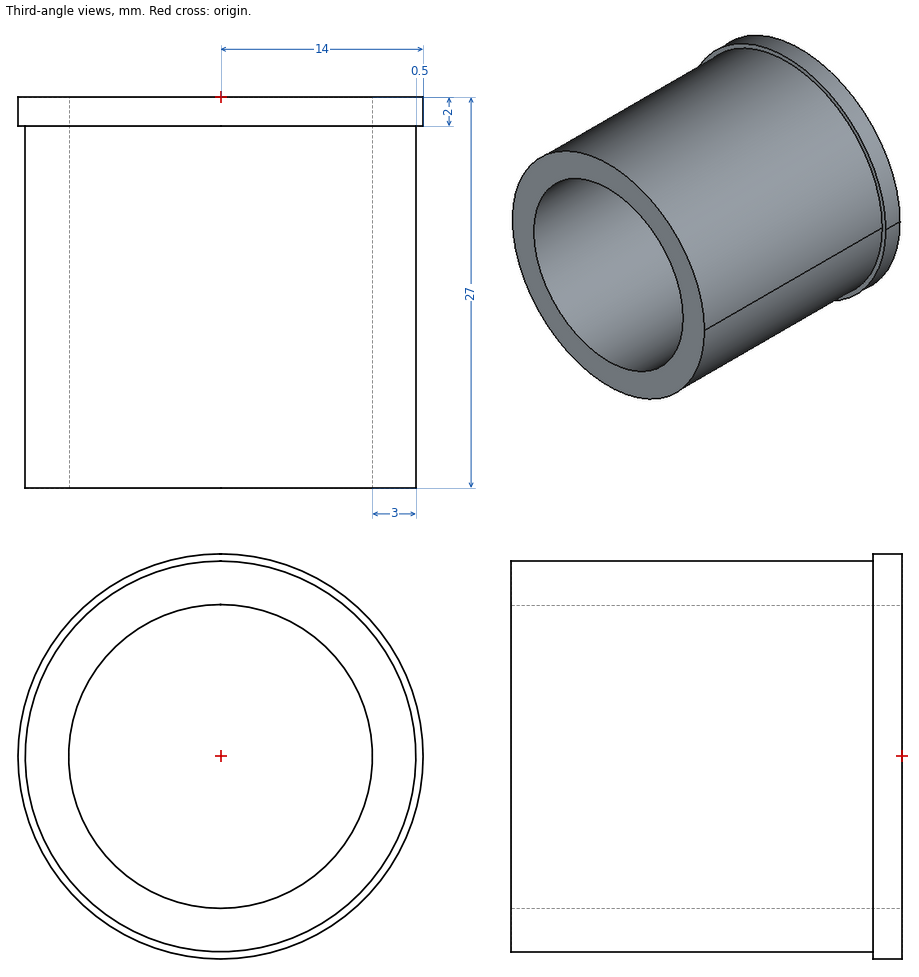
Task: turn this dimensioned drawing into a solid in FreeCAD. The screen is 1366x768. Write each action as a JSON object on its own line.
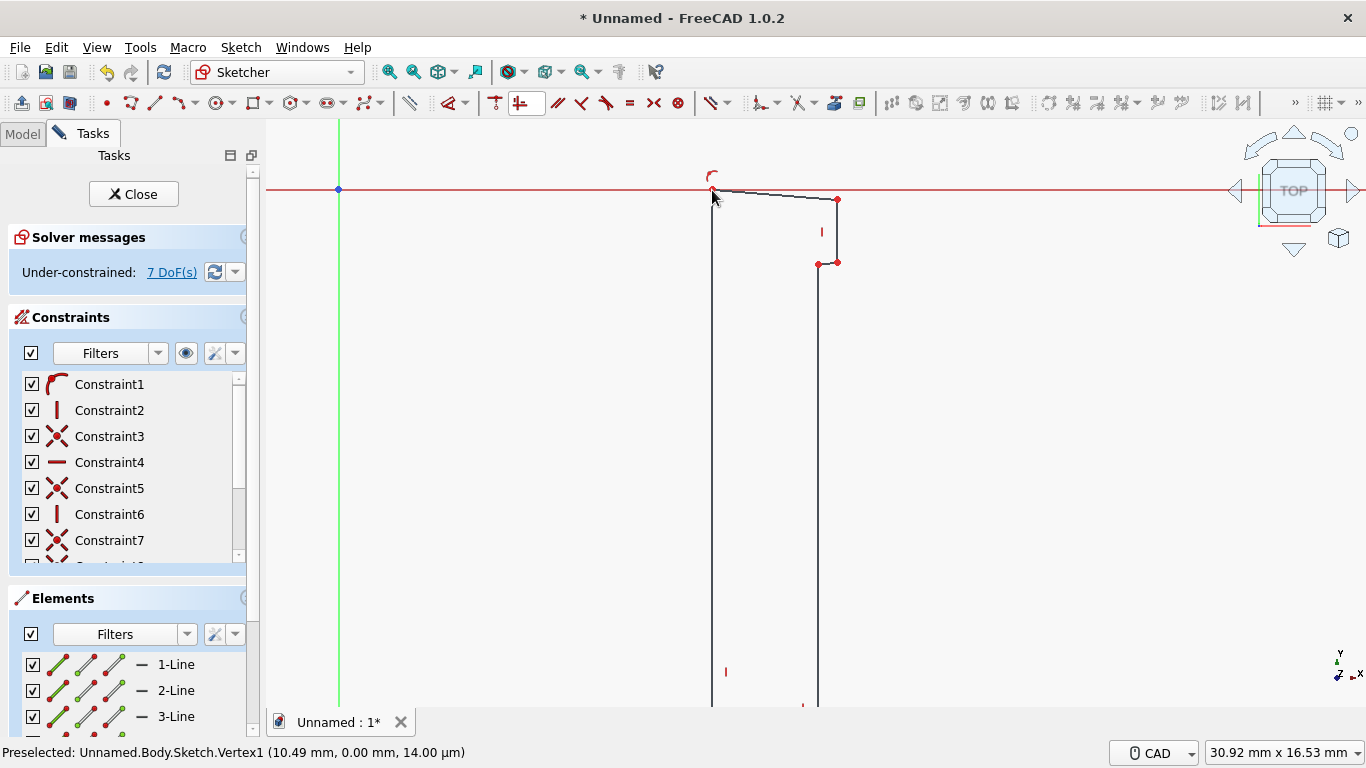
{"action": "scroll", "coordinate": [828, 264], "scroll_direction": "up", "scroll_amount": 2}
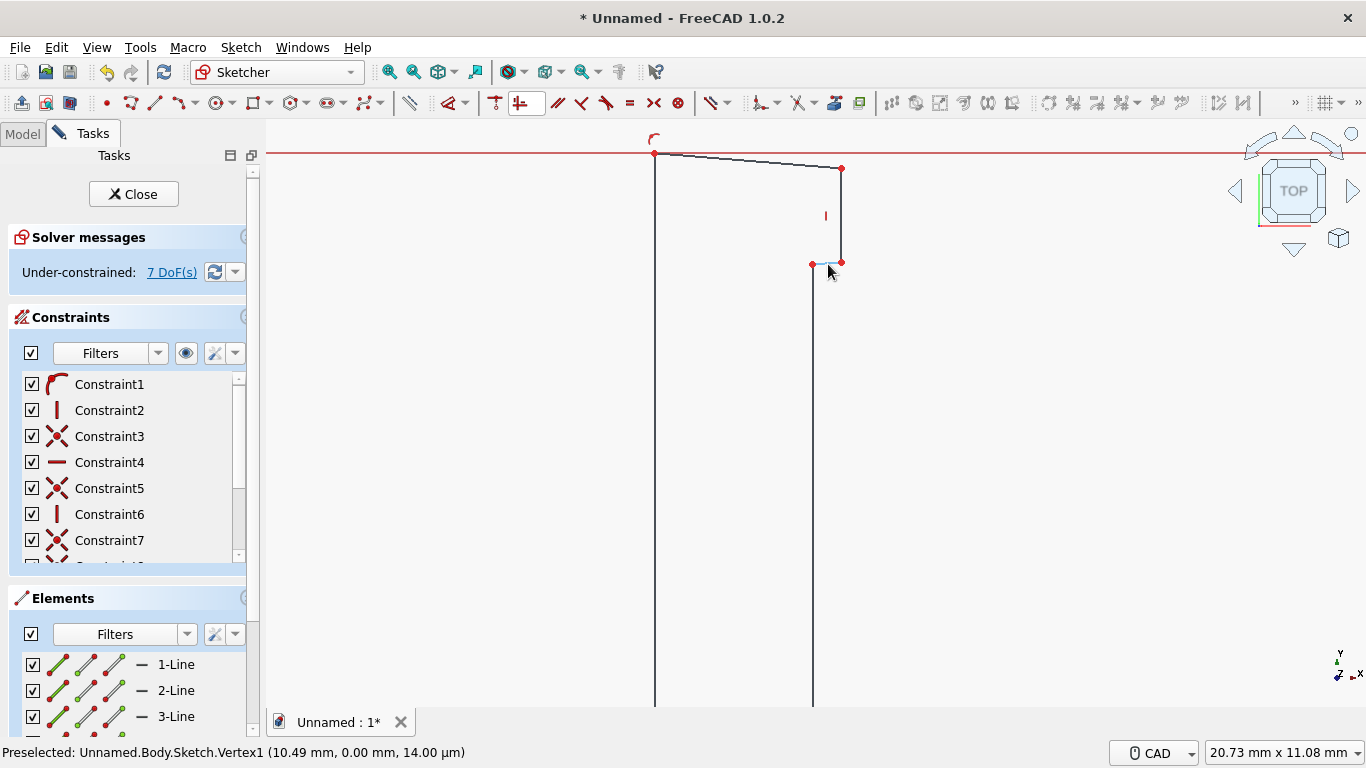
{"action": "left_click", "coordinate": [827, 263]}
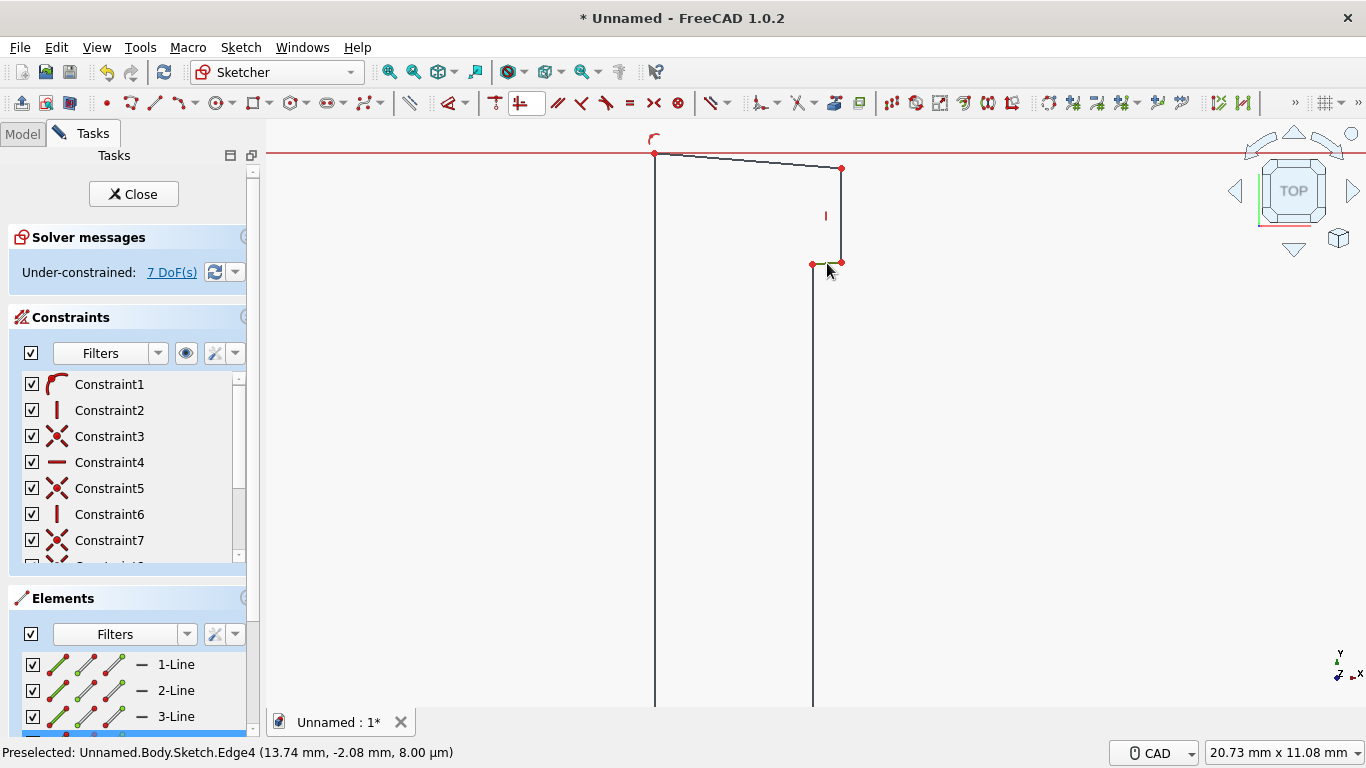
{"action": "key", "text": "h"}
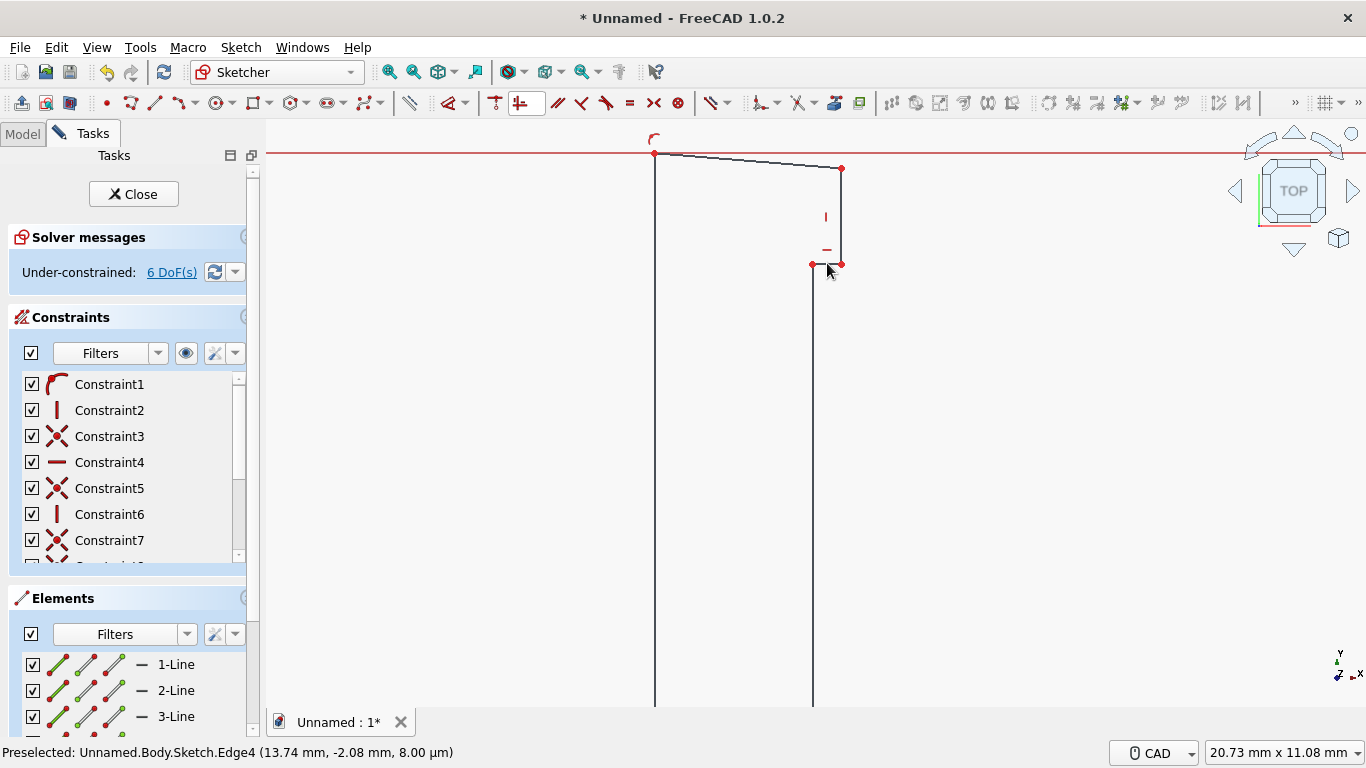
{"action": "scroll", "coordinate": [785, 164], "scroll_direction": "up", "scroll_amount": 2}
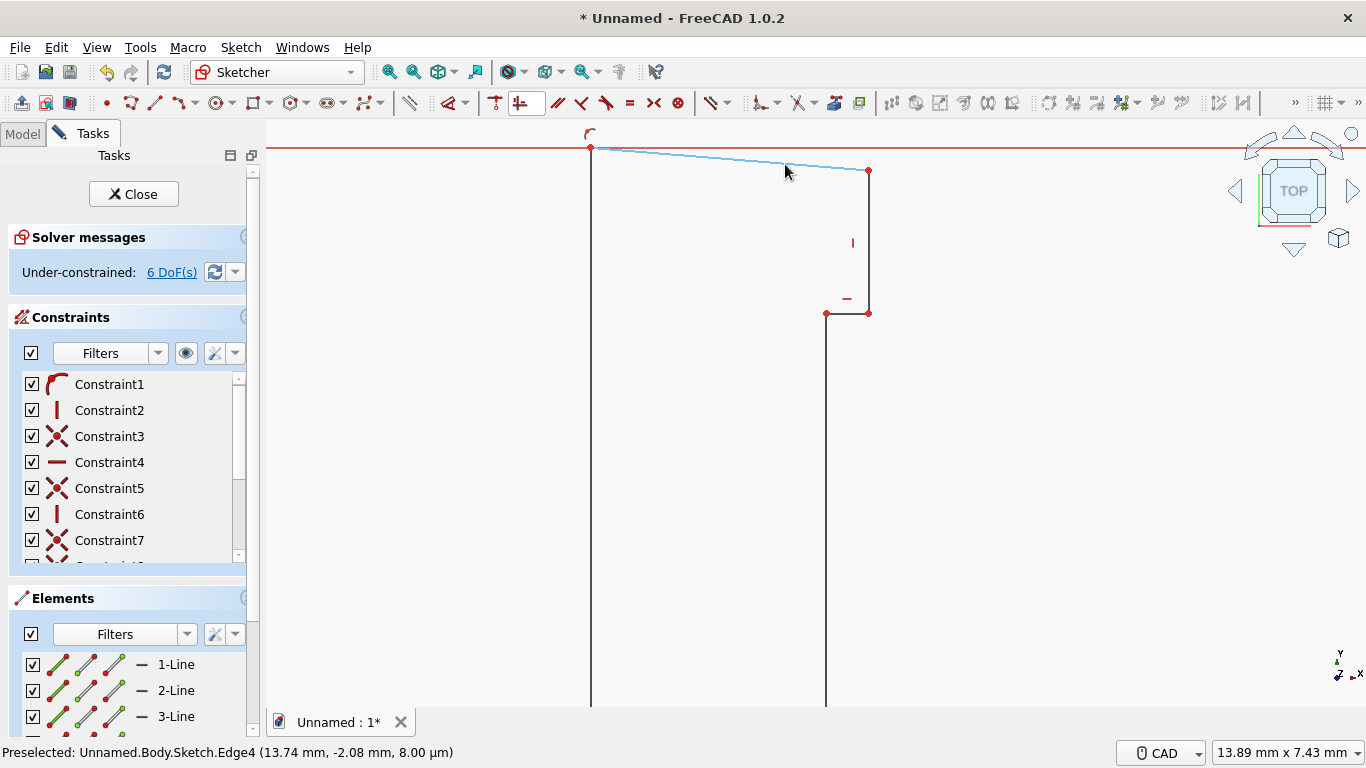
{"action": "left_click", "coordinate": [785, 164]}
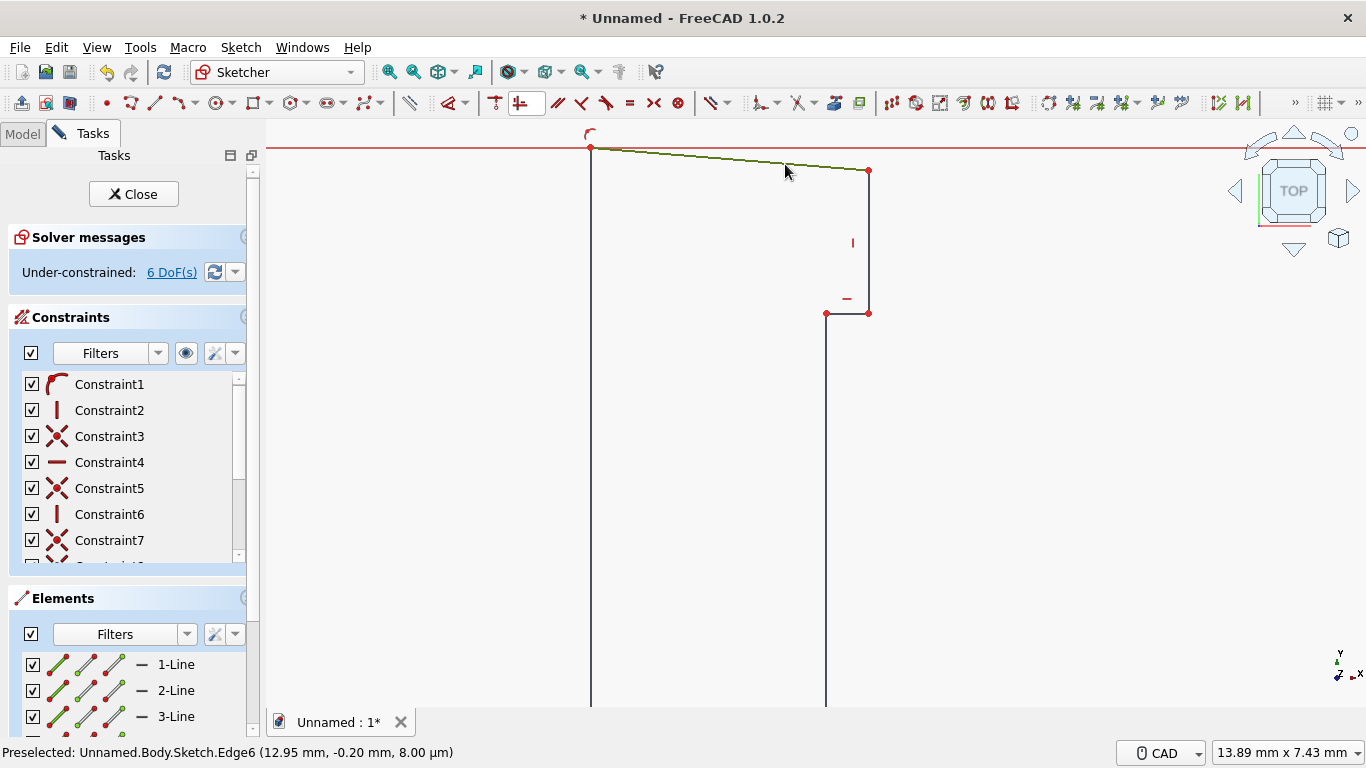
{"action": "key", "text": "h"}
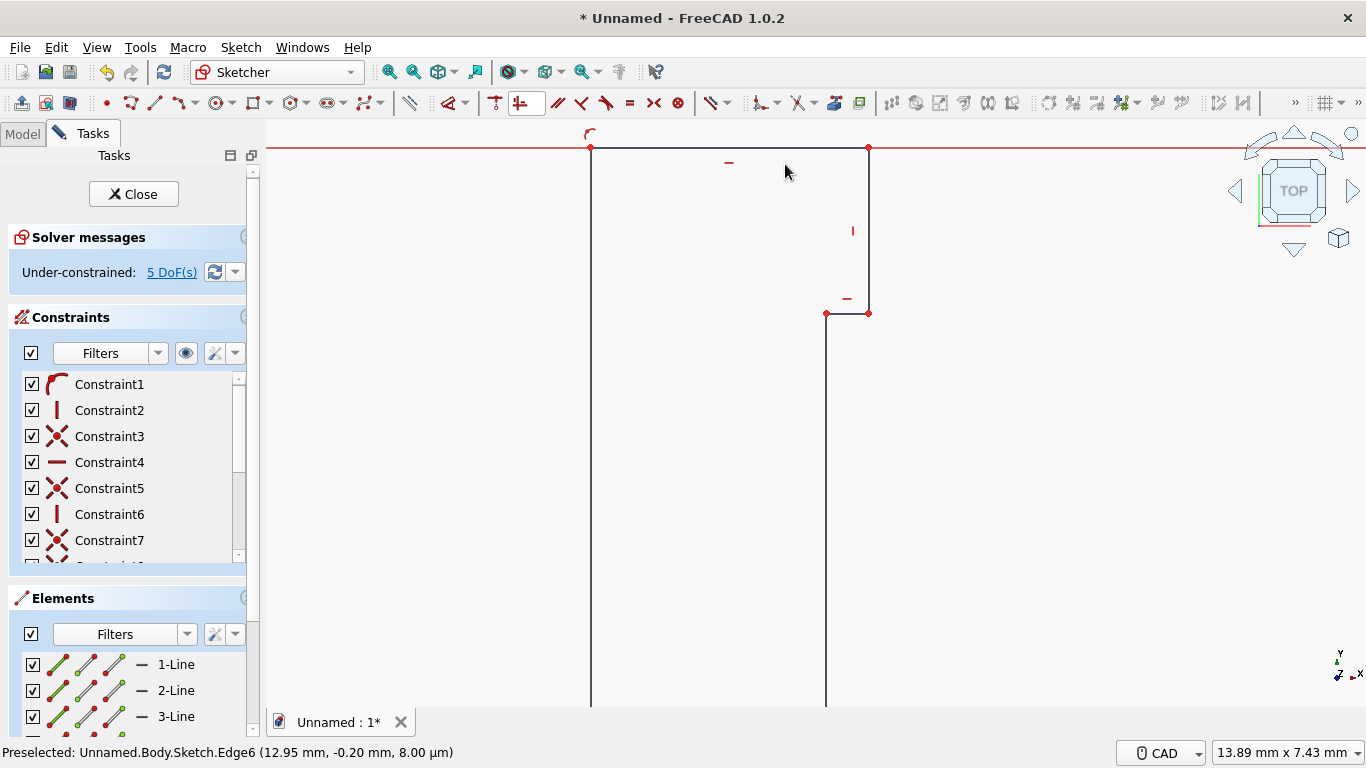
{"action": "scroll", "coordinate": [833, 254], "scroll_direction": "down", "scroll_amount": 9}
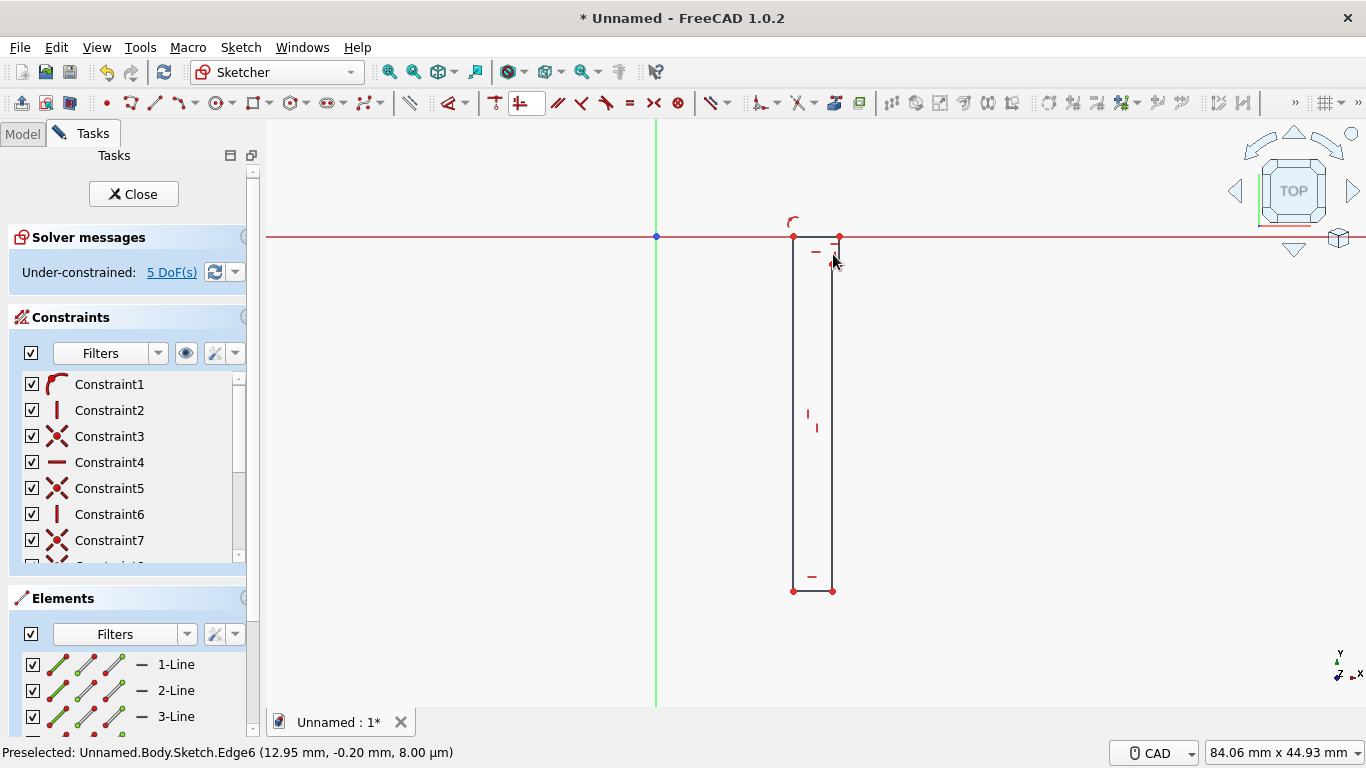
{"action": "left_click", "coordinate": [805, 591]}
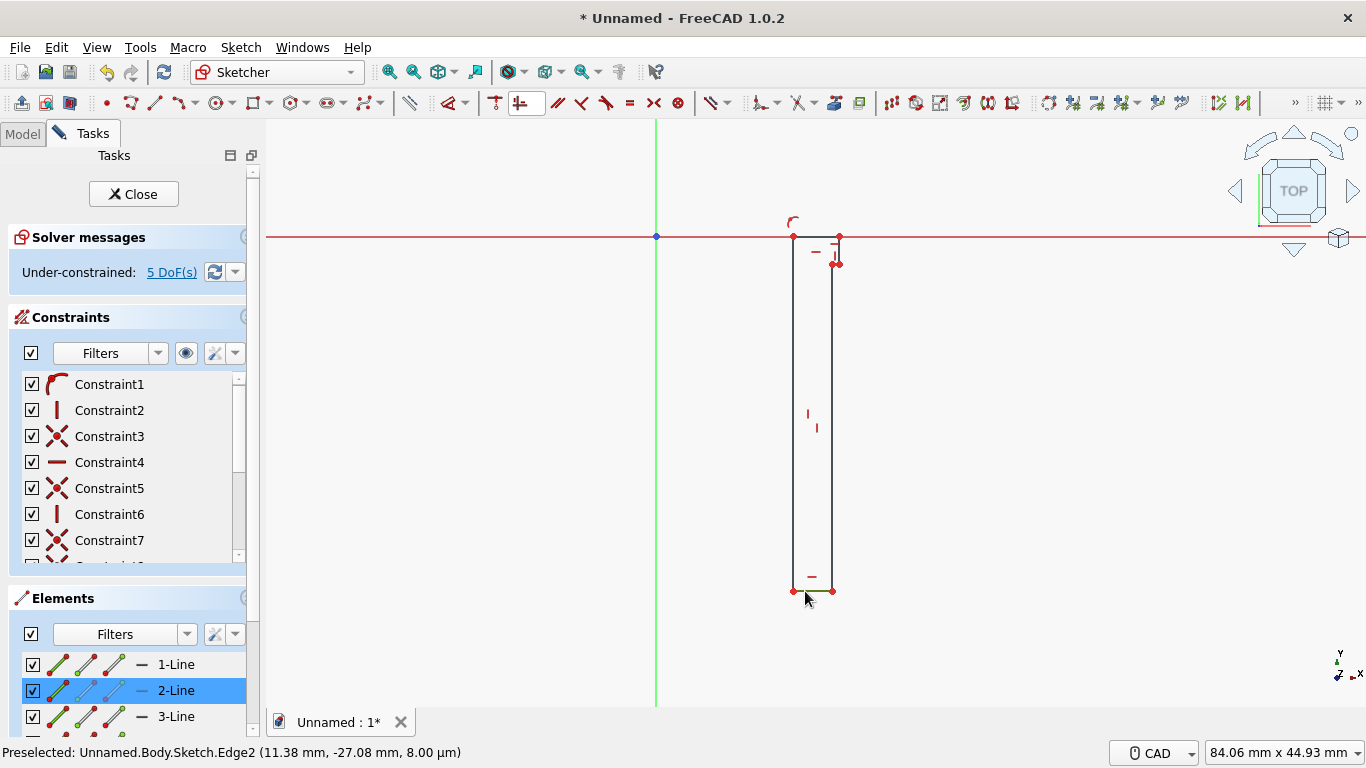
{"action": "key", "text": "l"}